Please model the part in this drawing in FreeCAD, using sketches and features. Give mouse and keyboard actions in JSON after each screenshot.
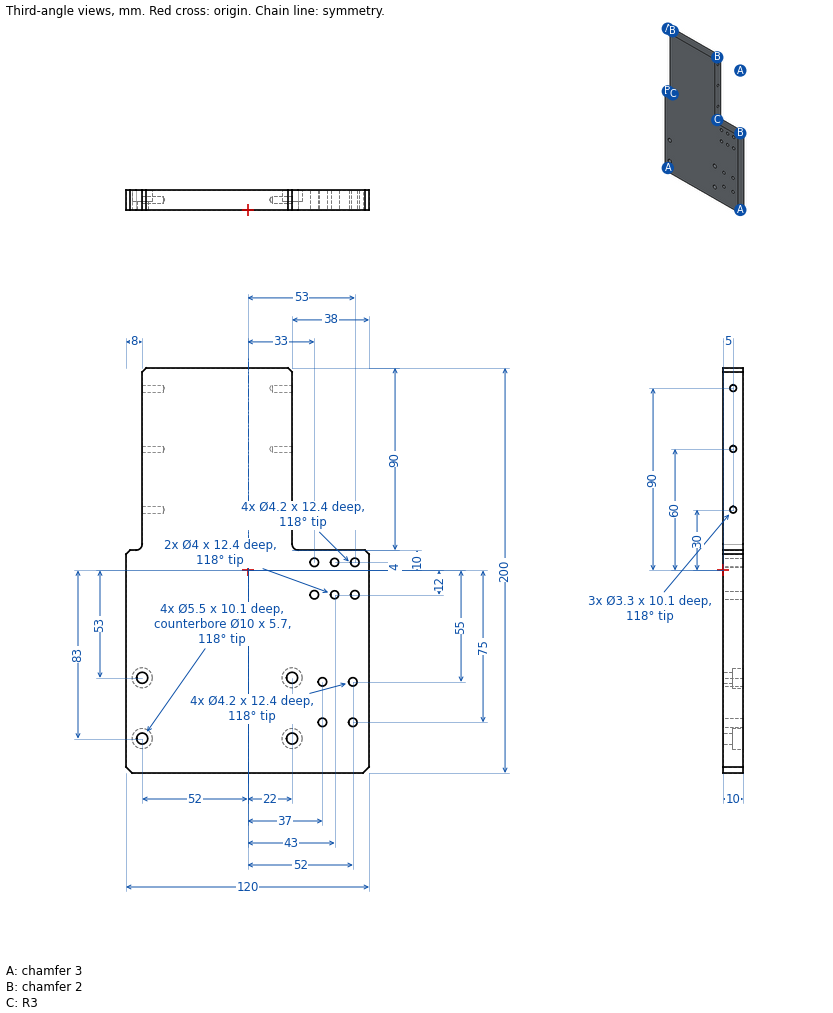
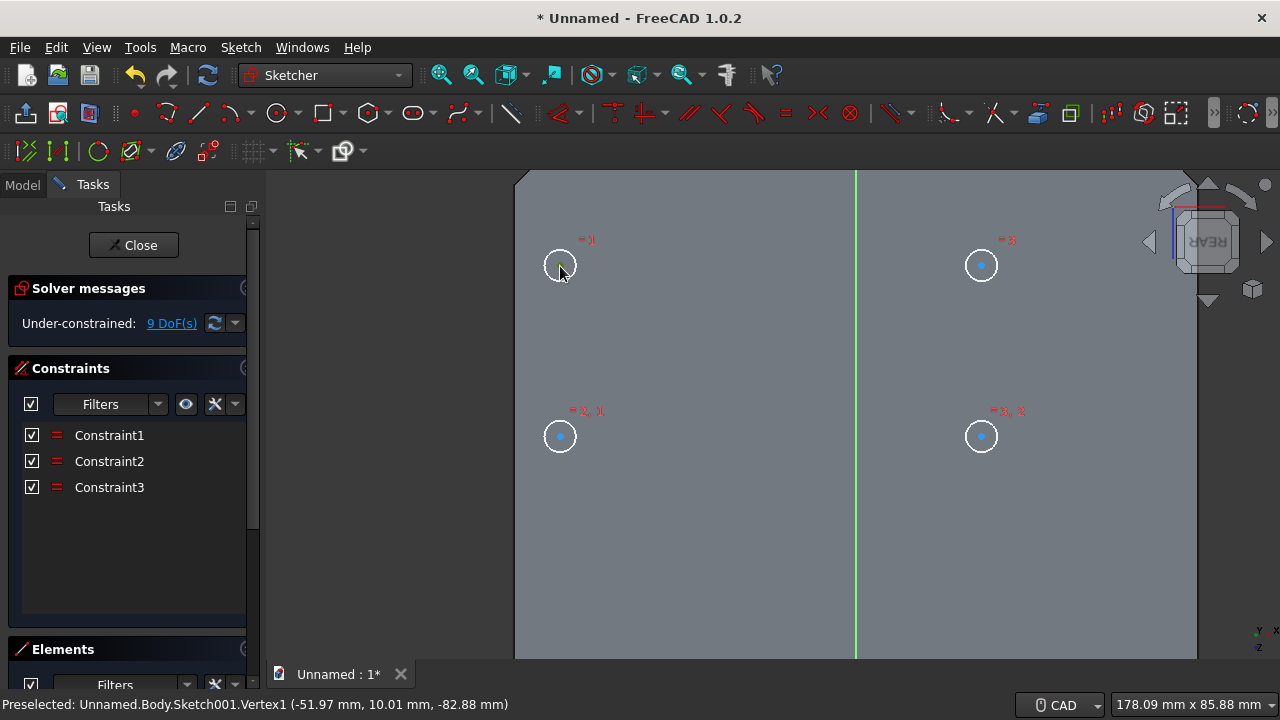
{"action": "left_click", "coordinate": [560, 436]}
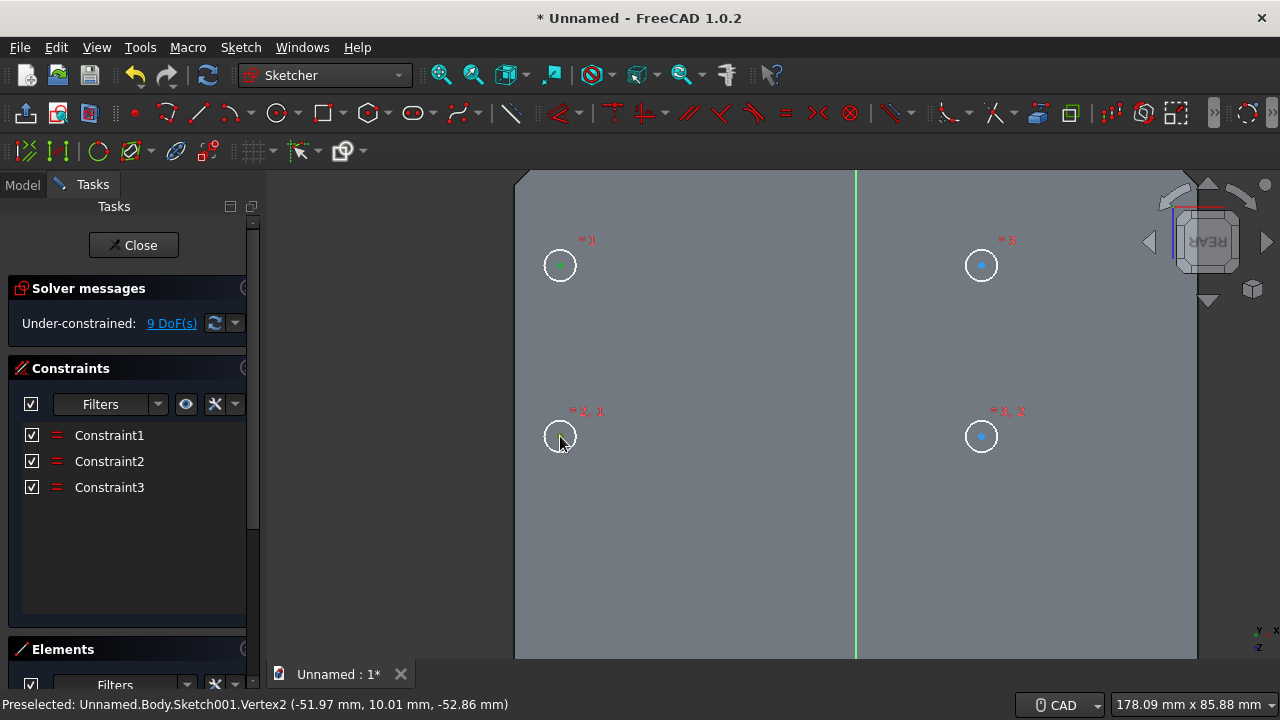
{"action": "left_click", "coordinate": [668, 114]}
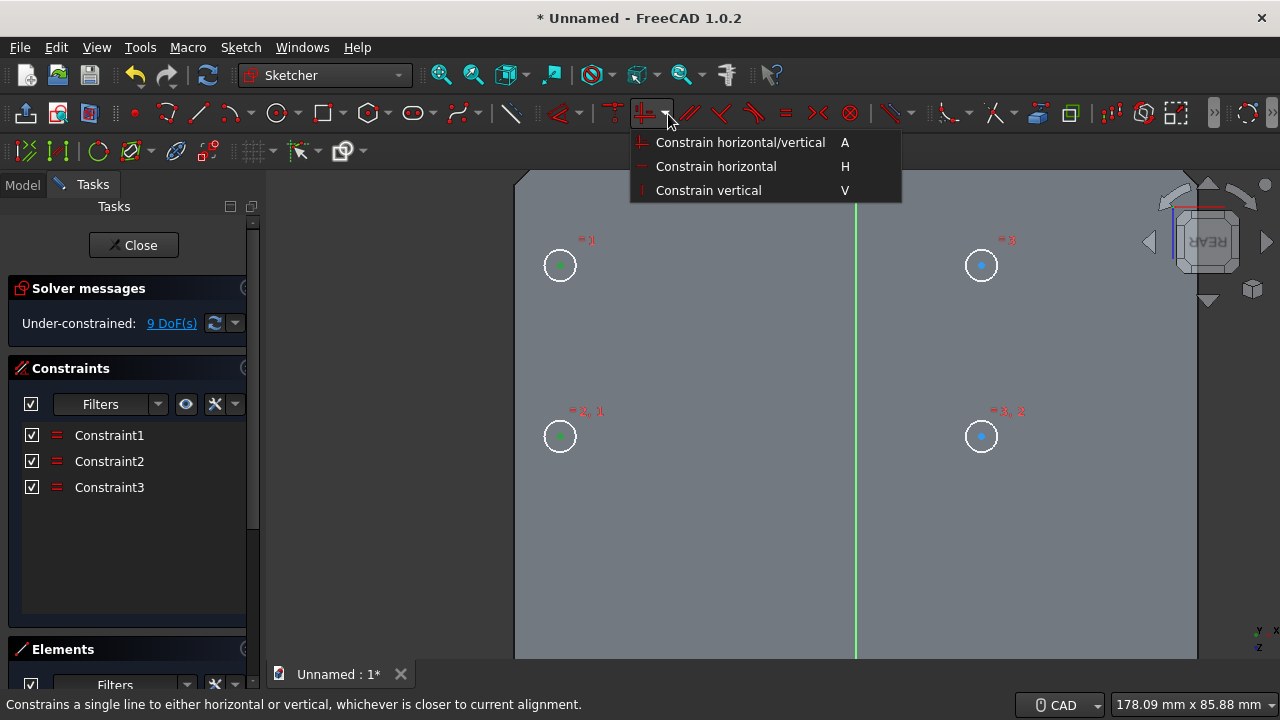
{"action": "left_click", "coordinate": [766, 190]}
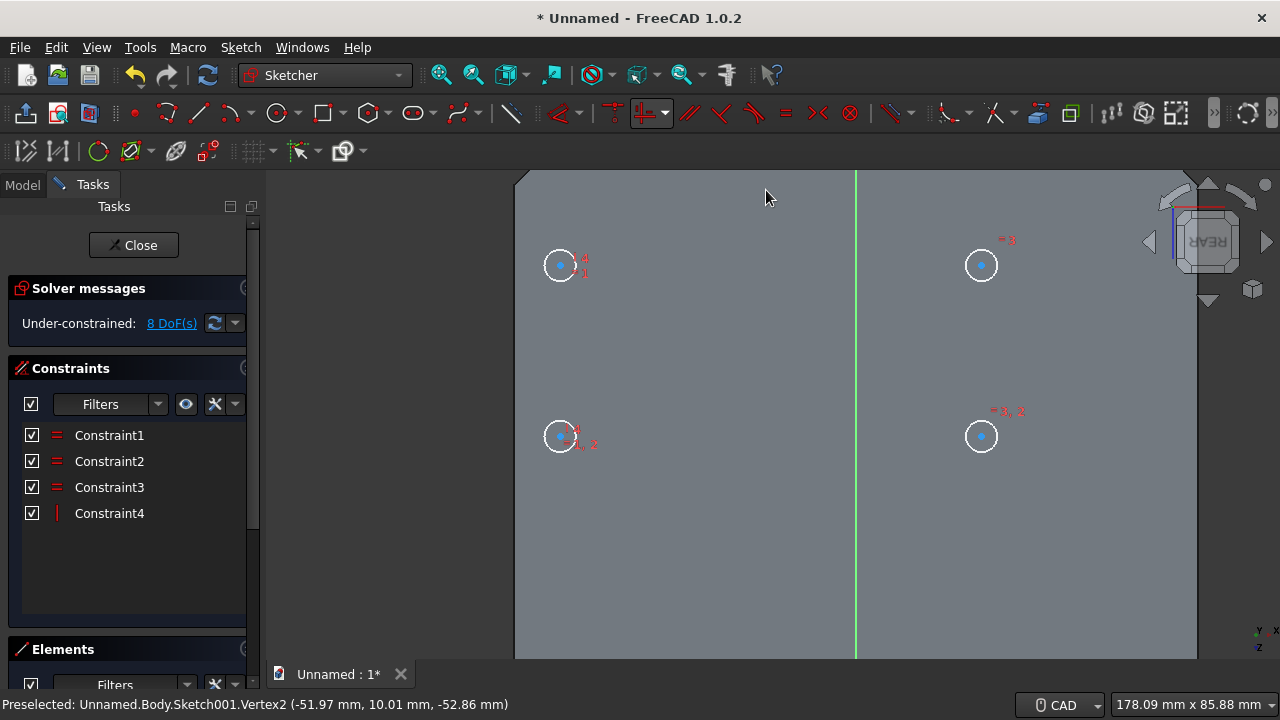
{"action": "left_click", "coordinate": [560, 436]}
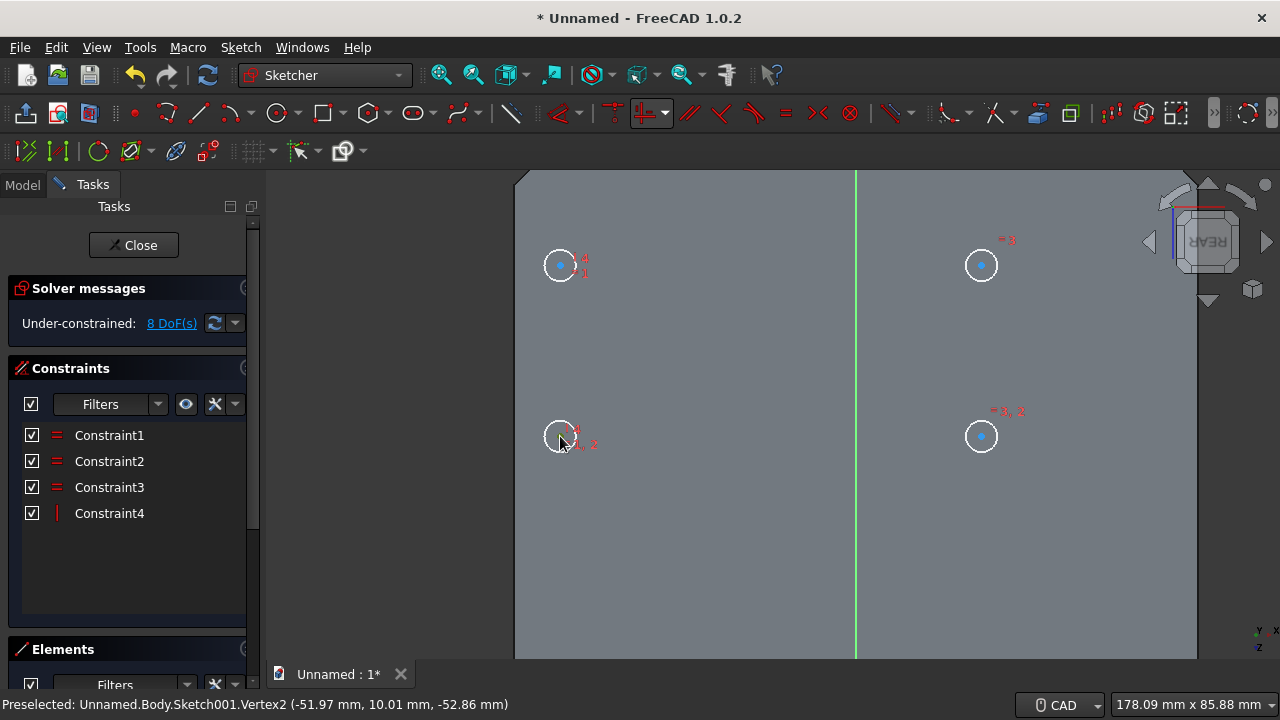
{"action": "left_click", "coordinate": [982, 436]}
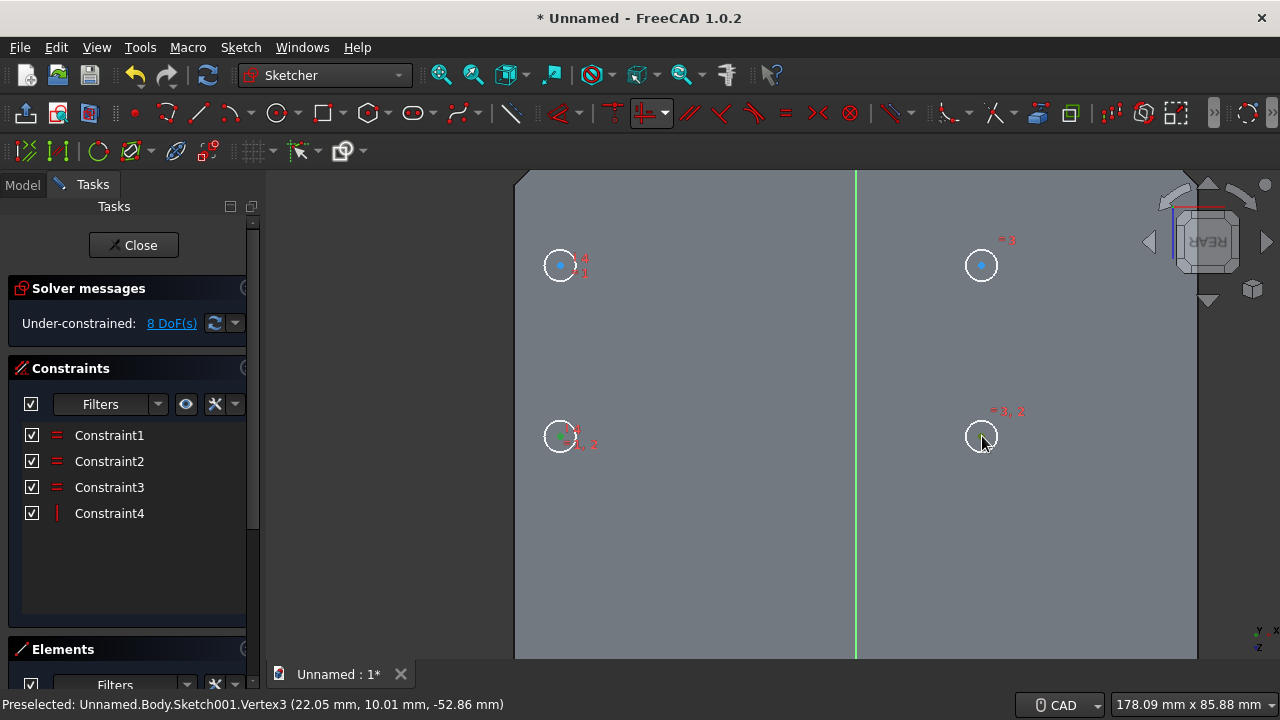
{"action": "left_click", "coordinate": [668, 114]}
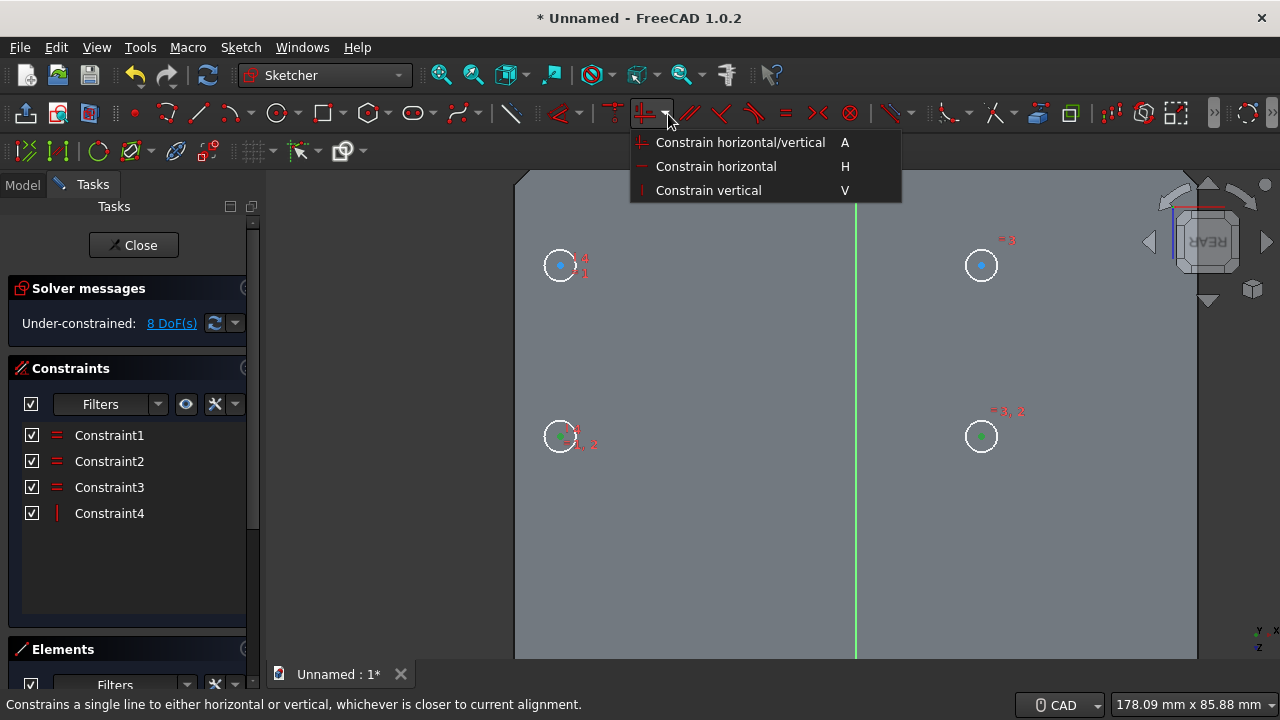
{"action": "left_click", "coordinate": [766, 166]}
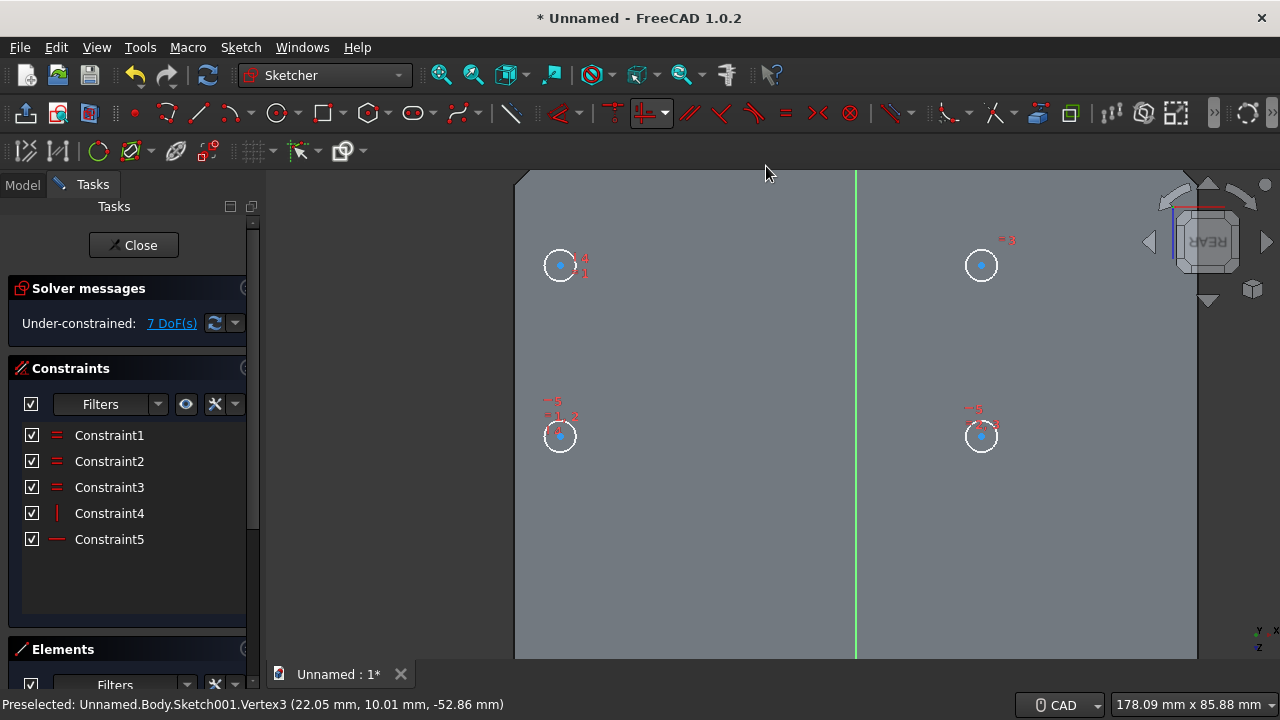
{"action": "left_click", "coordinate": [982, 436]}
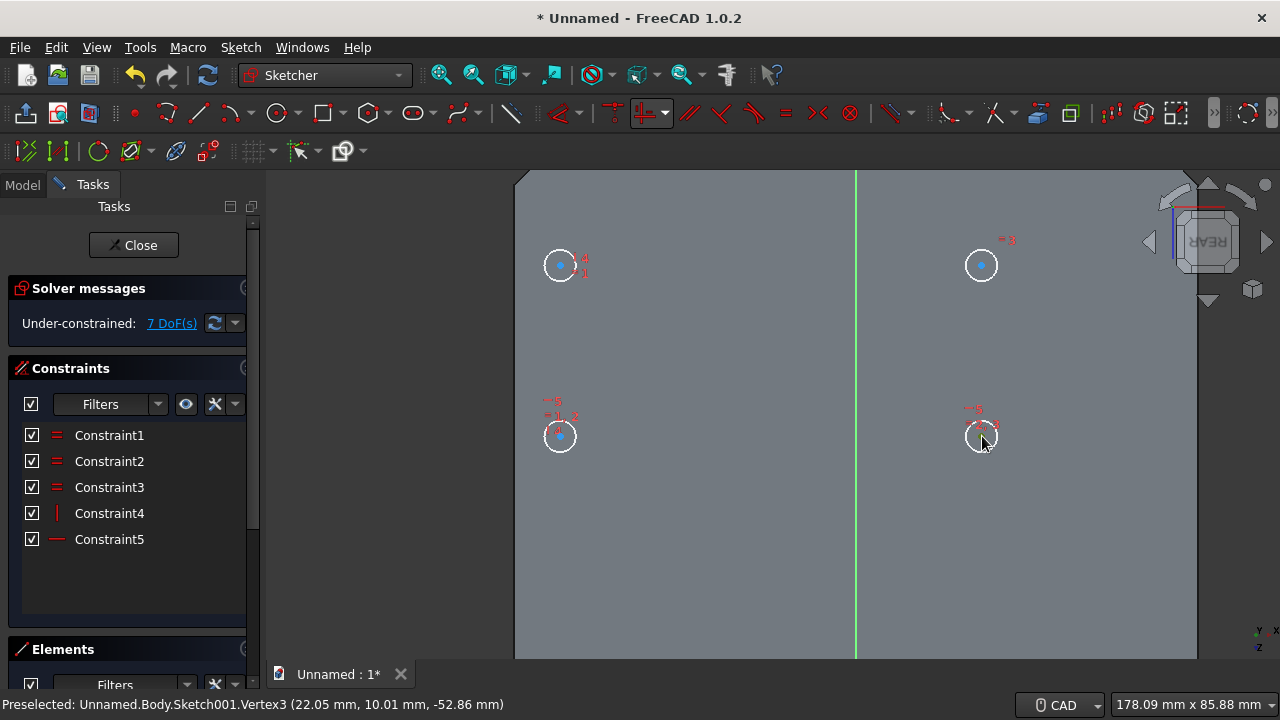
{"action": "left_click", "coordinate": [982, 266]}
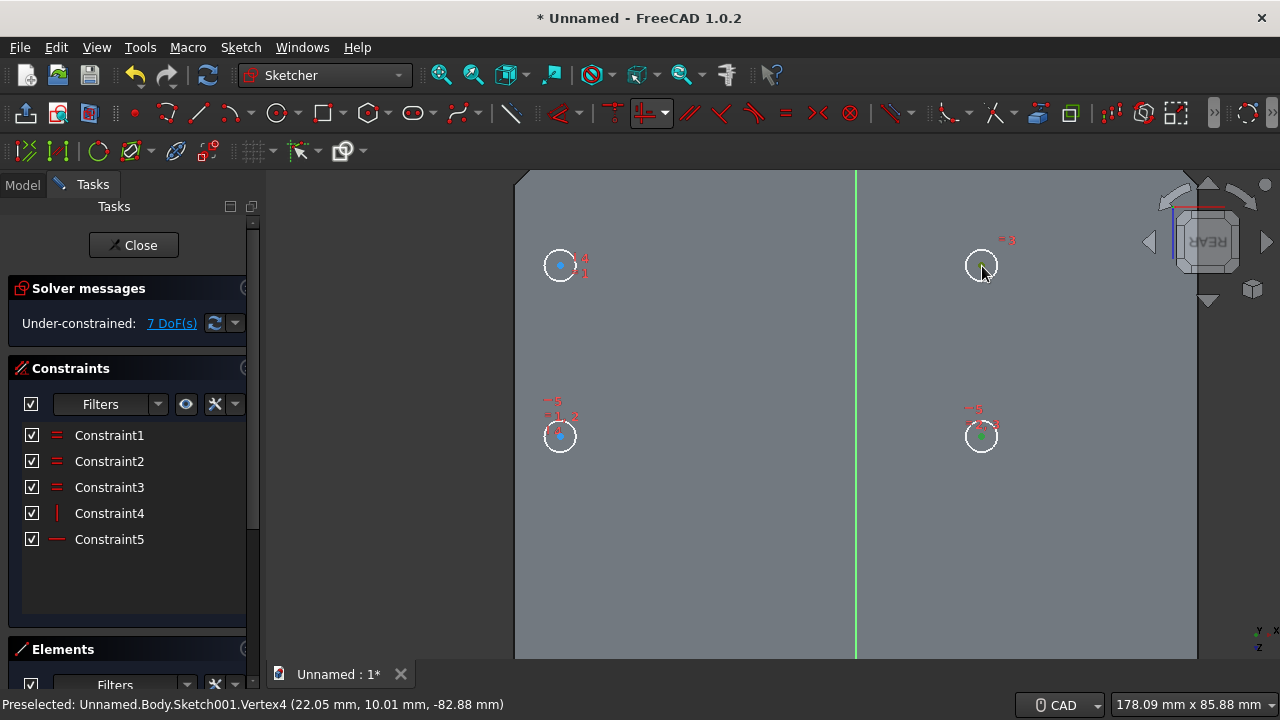
{"action": "left_click", "coordinate": [668, 114]}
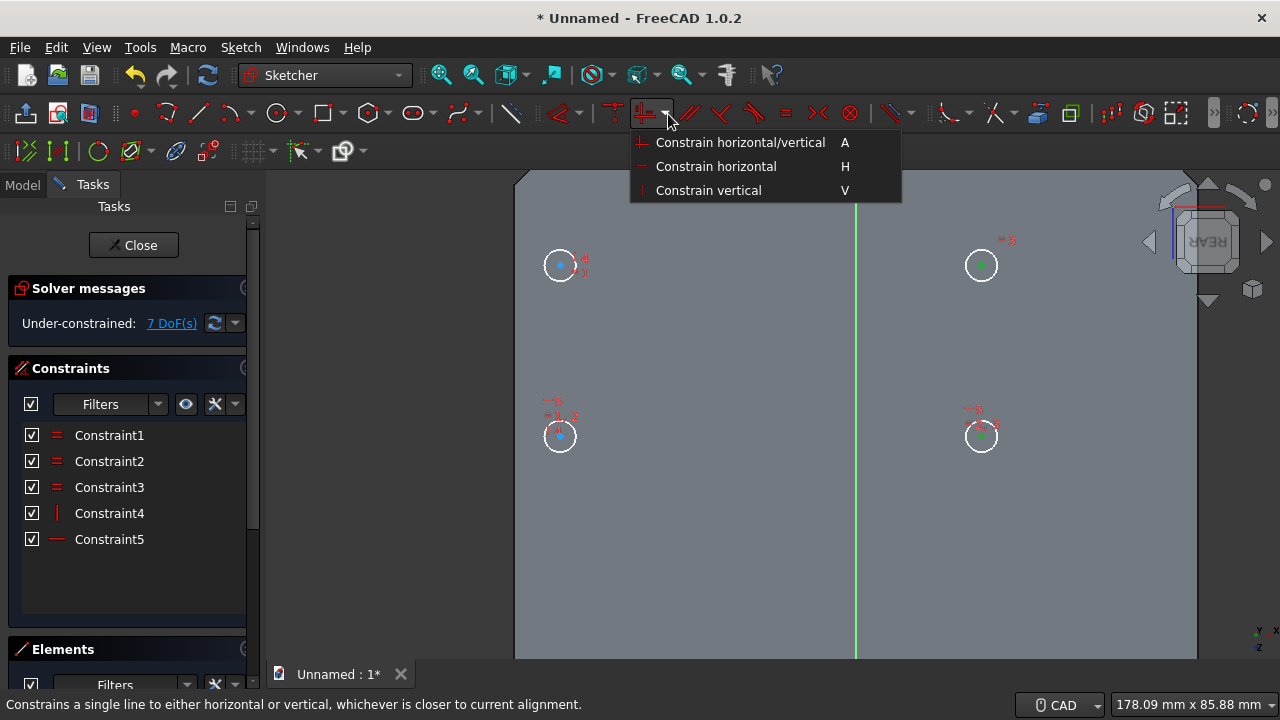
{"action": "left_click", "coordinate": [766, 190]}